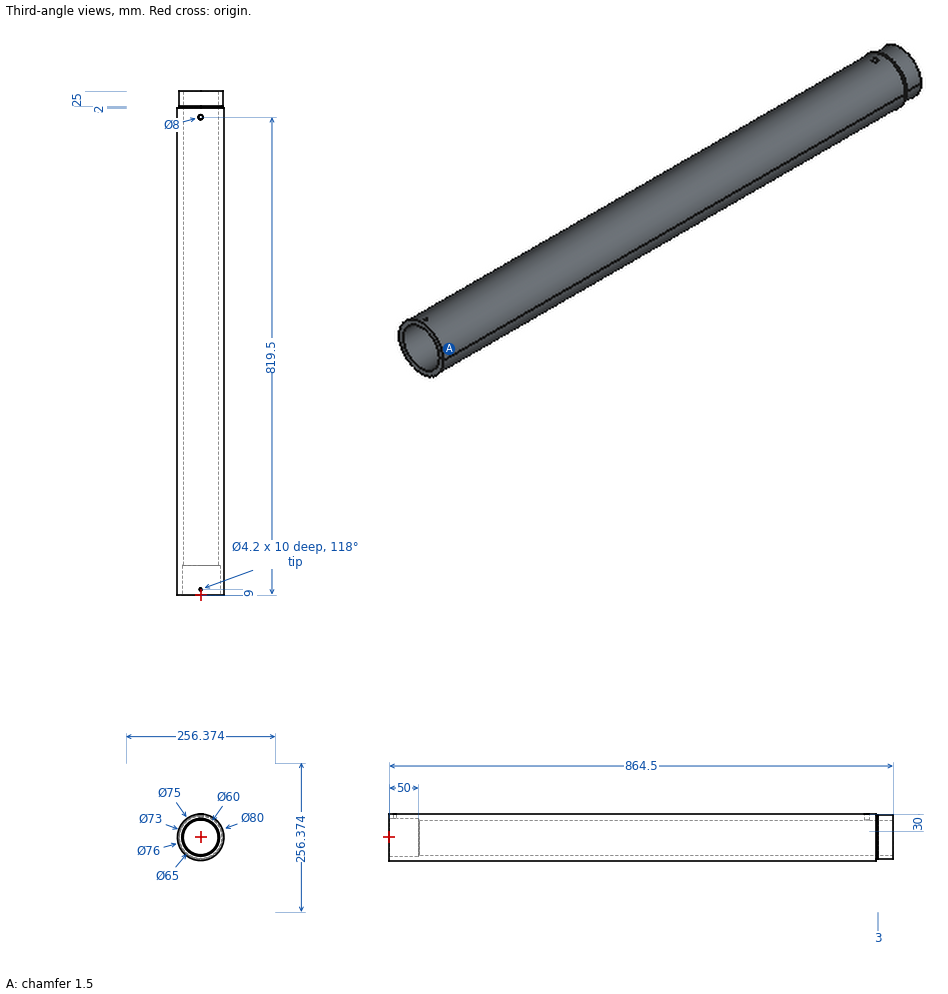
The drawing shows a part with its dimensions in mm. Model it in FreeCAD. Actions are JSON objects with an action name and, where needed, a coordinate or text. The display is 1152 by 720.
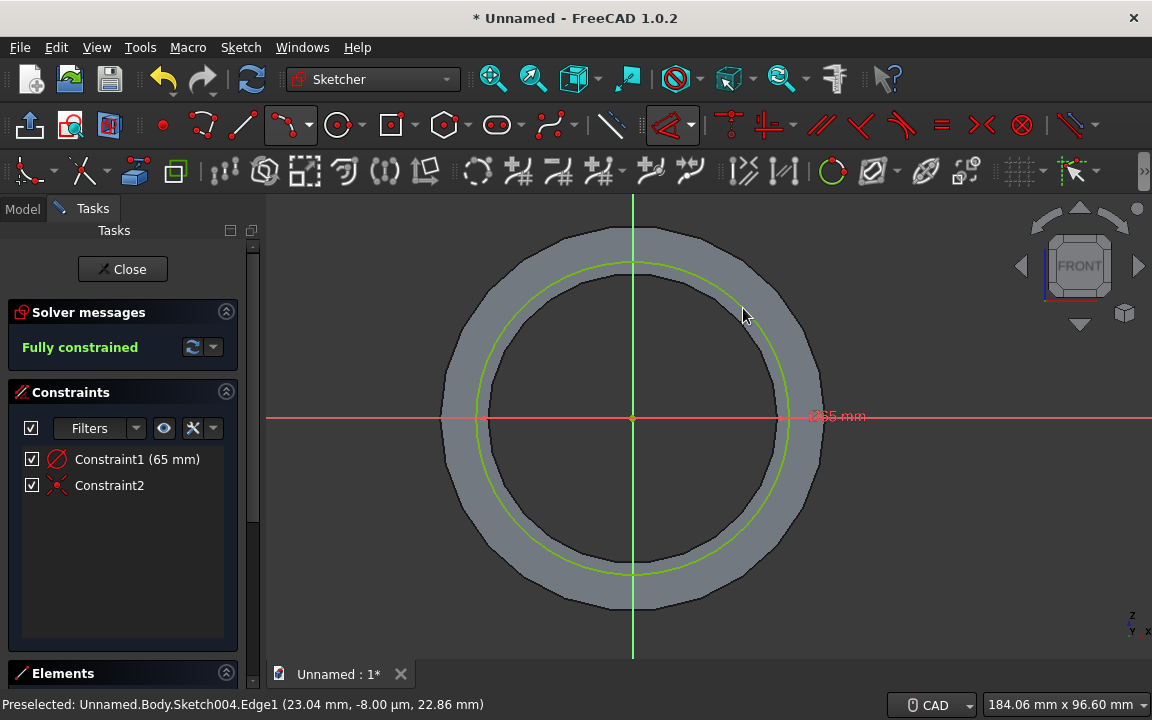
{"action": "left_click", "coordinate": [123, 269]}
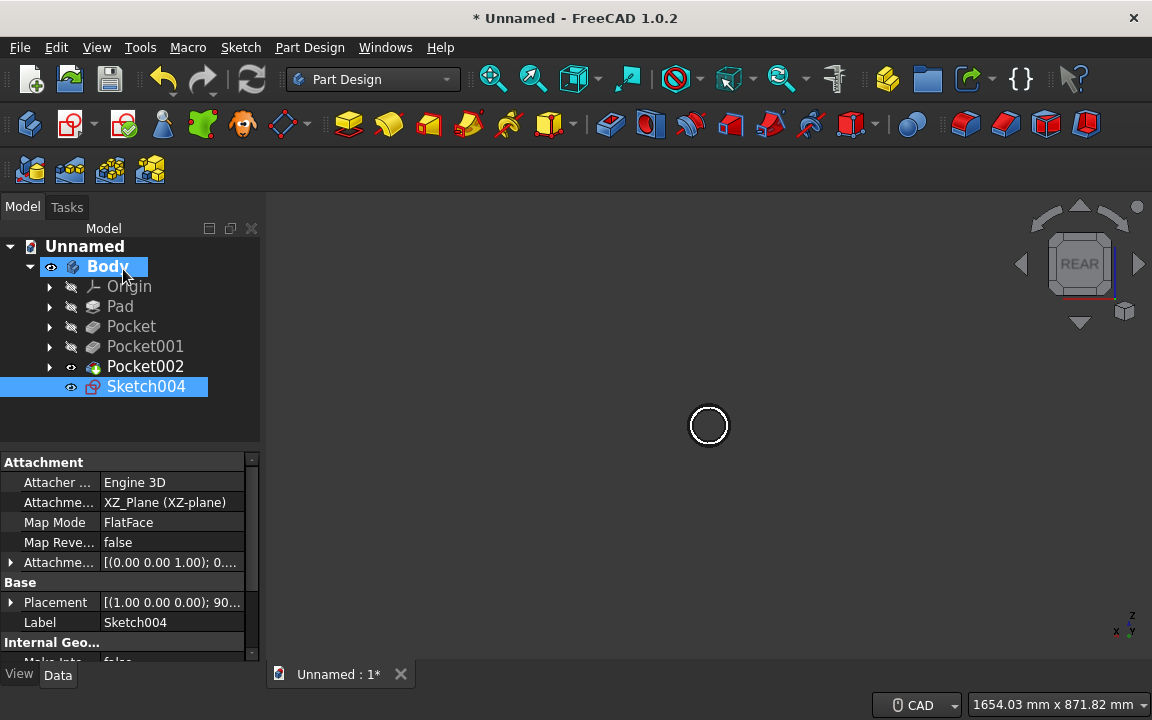
{"action": "left_click", "coordinate": [612, 124]}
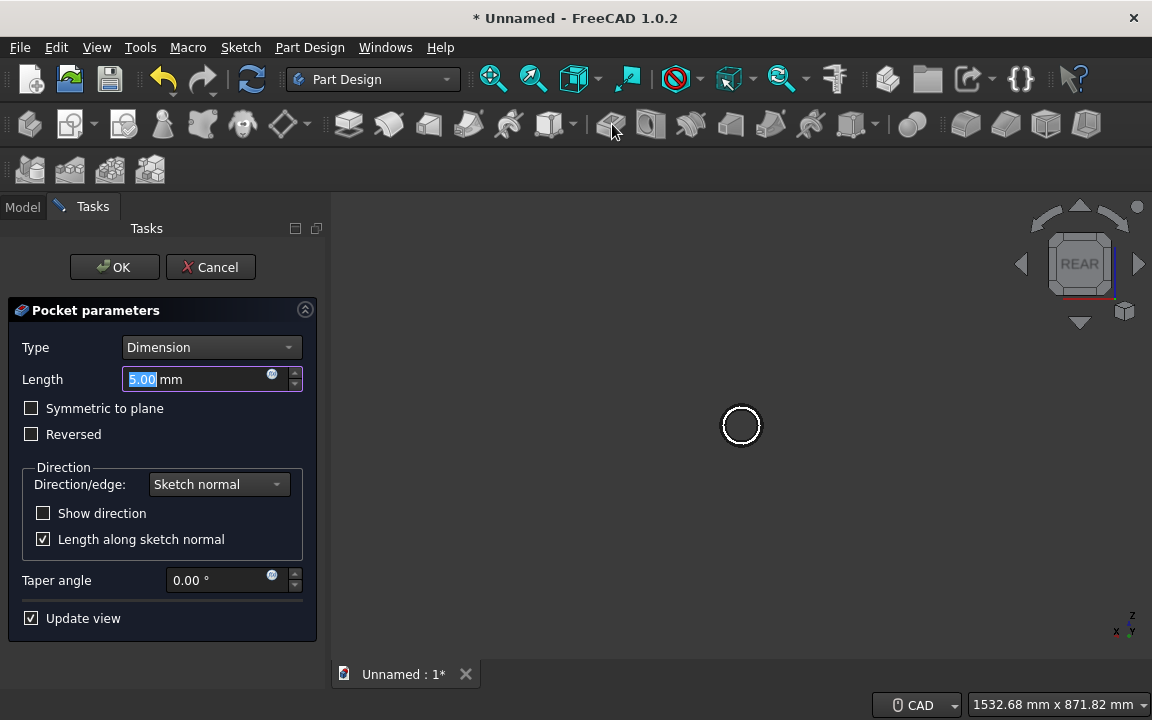
{"action": "type", "text": "50"}
{"action": "key", "text": "Tab"}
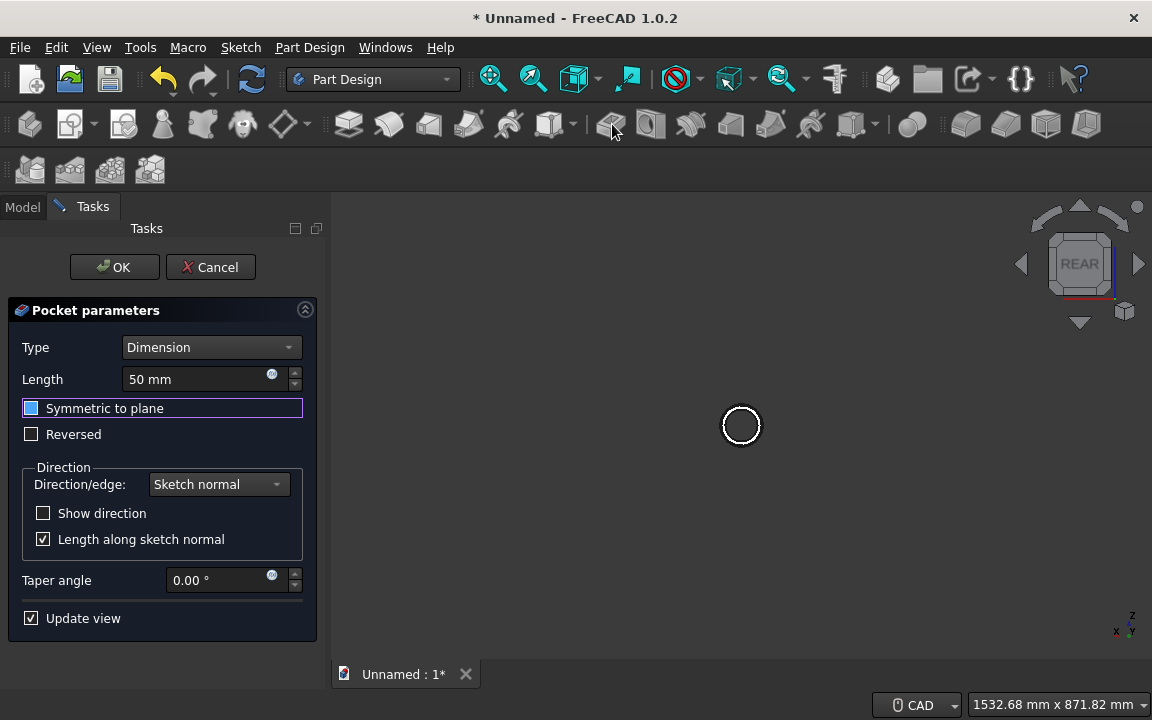
{"action": "left_click", "coordinate": [115, 267]}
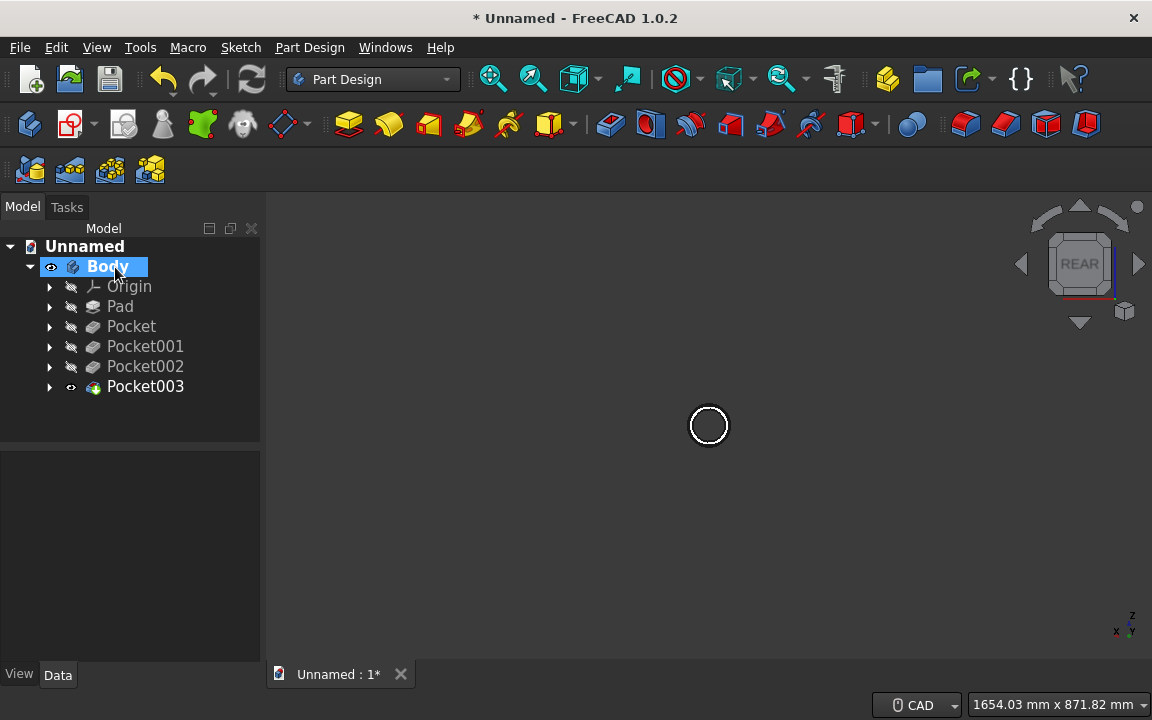
{"action": "left_click", "coordinate": [494, 80]}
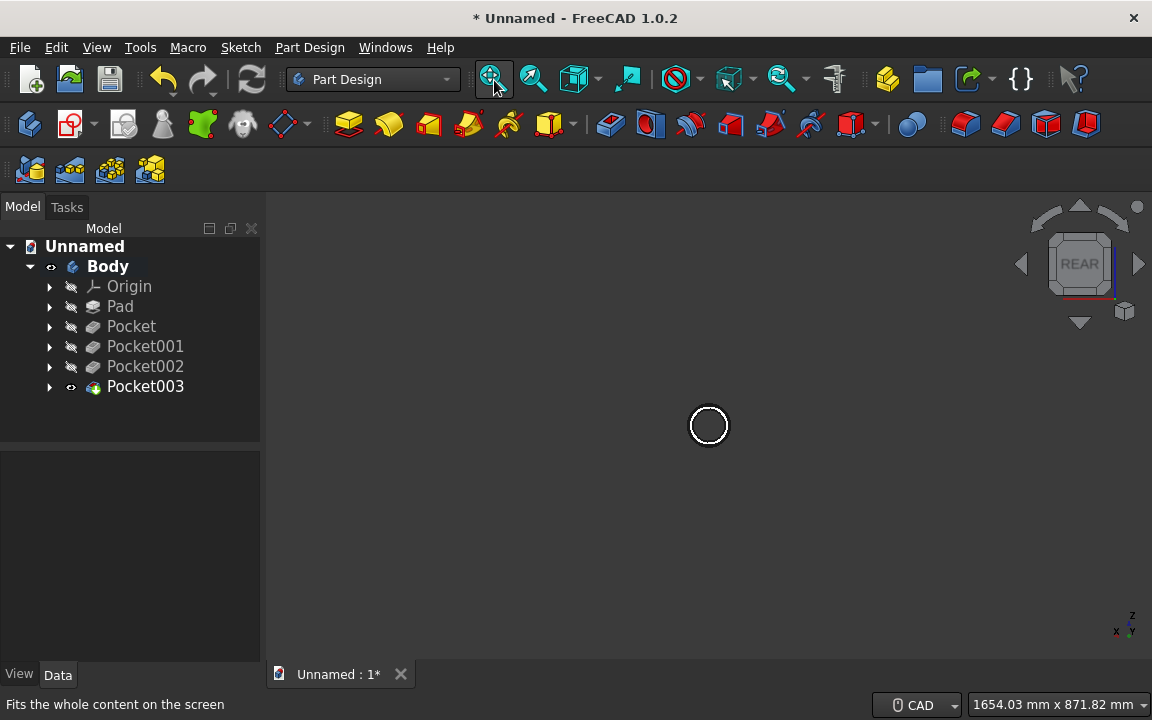
{"action": "key", "text": "0"}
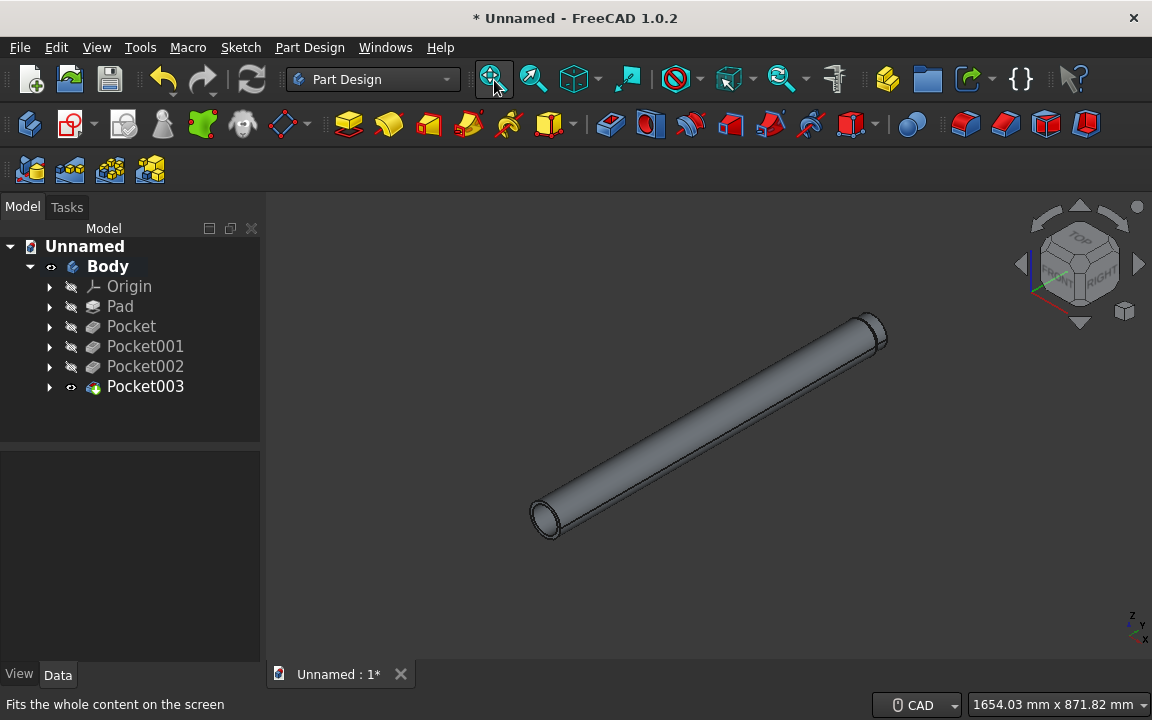
{"action": "key", "text": "2"}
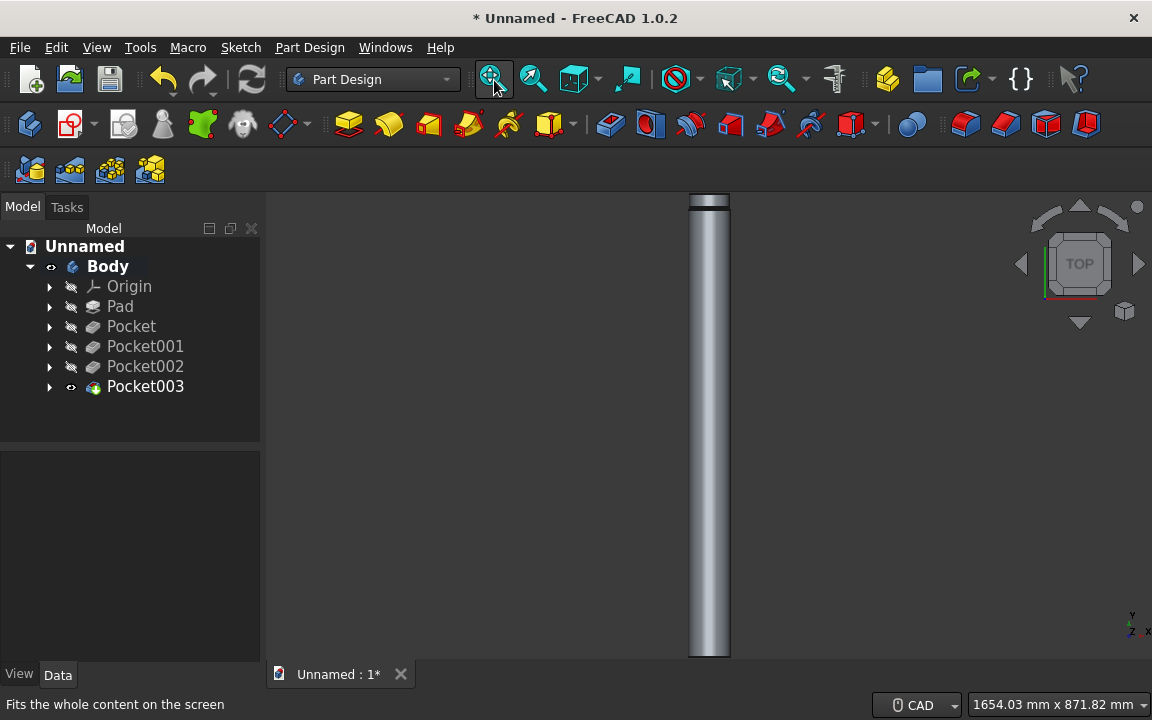
{"action": "key", "text": "1"}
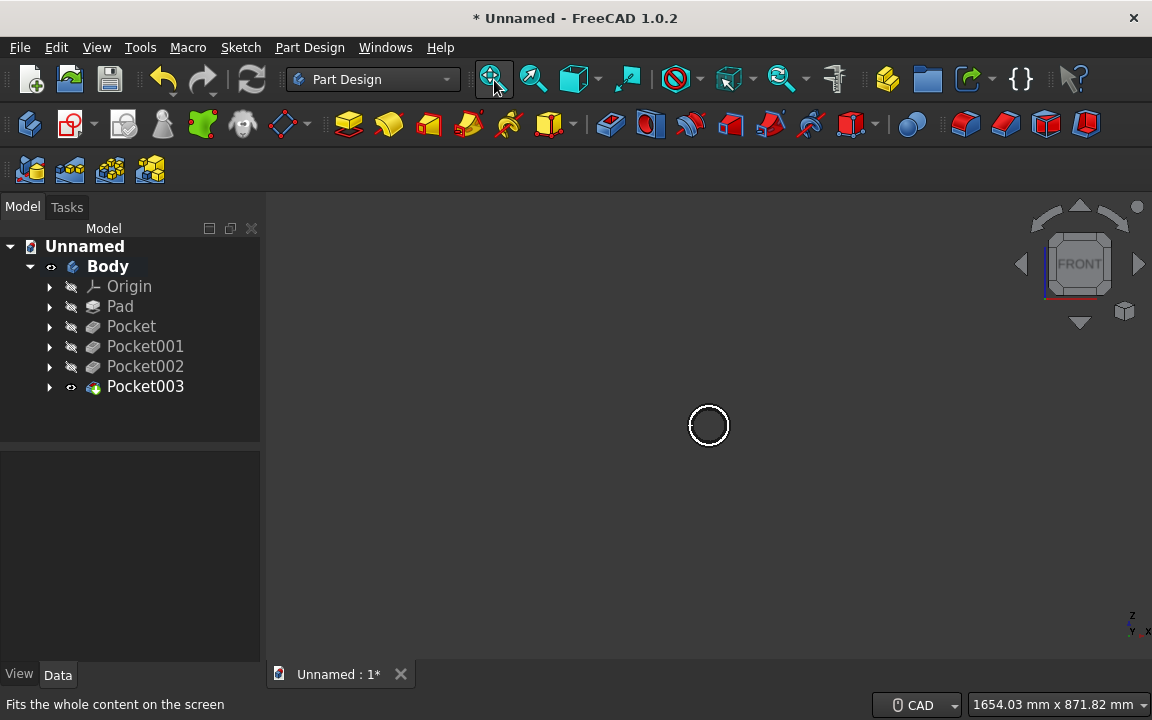
{"action": "left_click", "coordinate": [494, 80]}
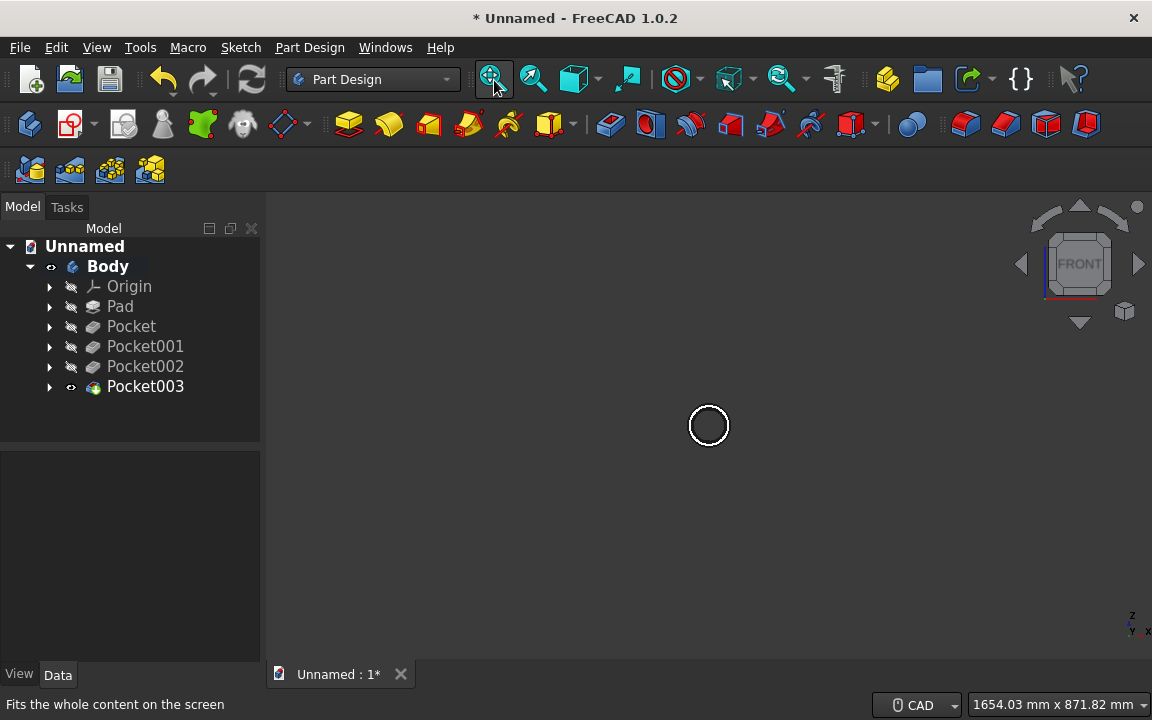
{"action": "key", "text": "3"}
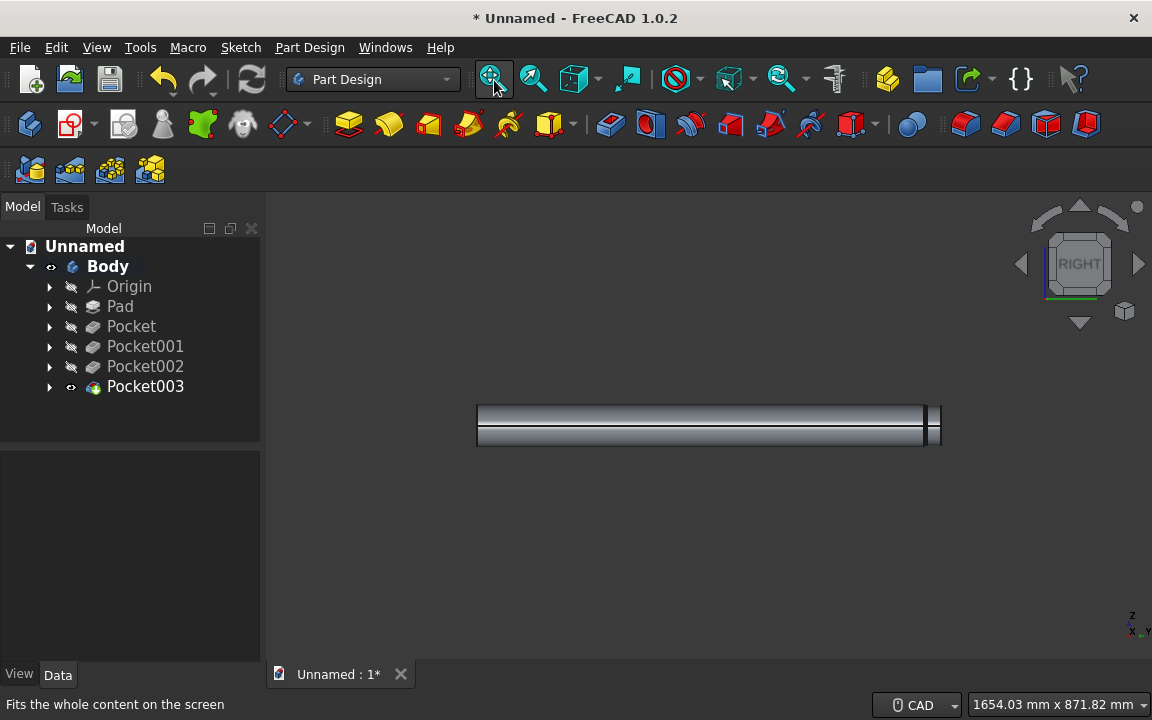
{"action": "key", "text": "5"}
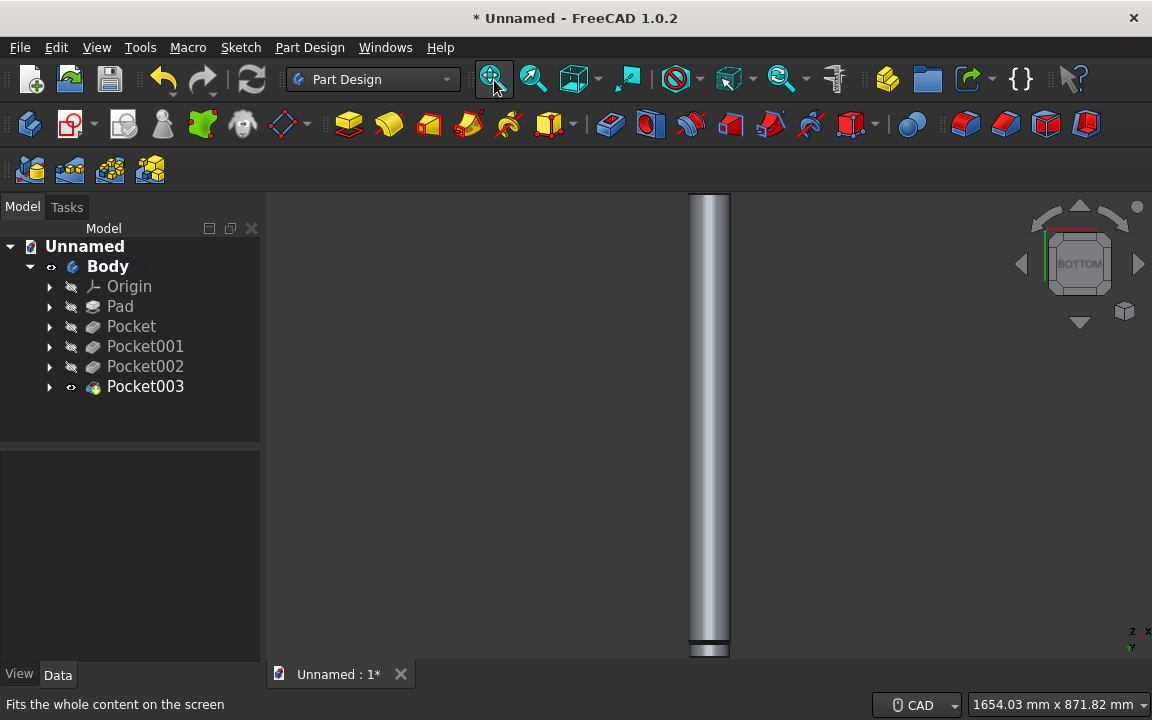
{"action": "key", "text": "4"}